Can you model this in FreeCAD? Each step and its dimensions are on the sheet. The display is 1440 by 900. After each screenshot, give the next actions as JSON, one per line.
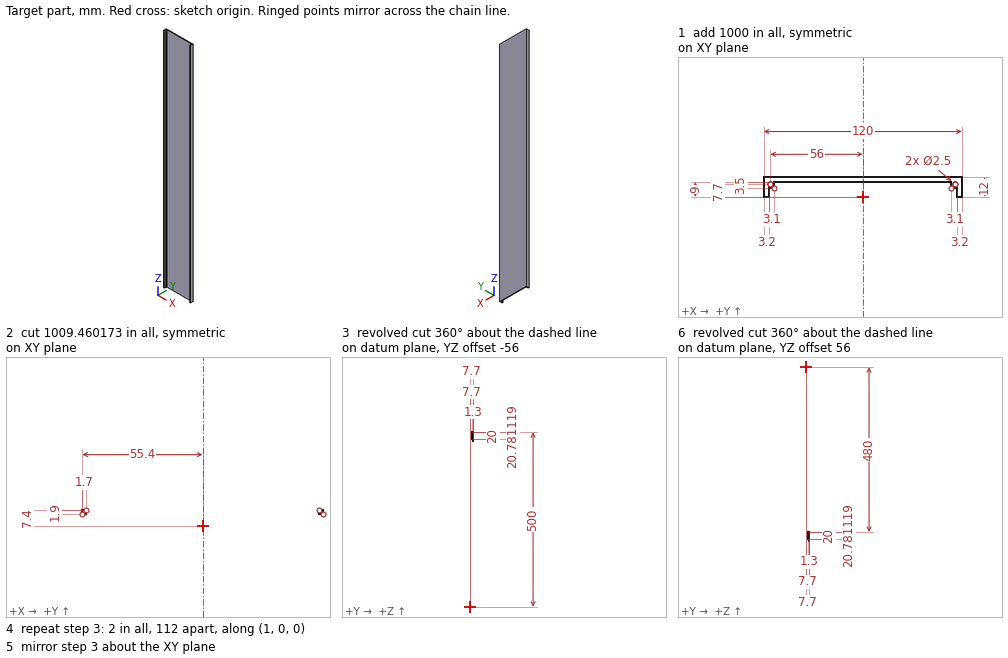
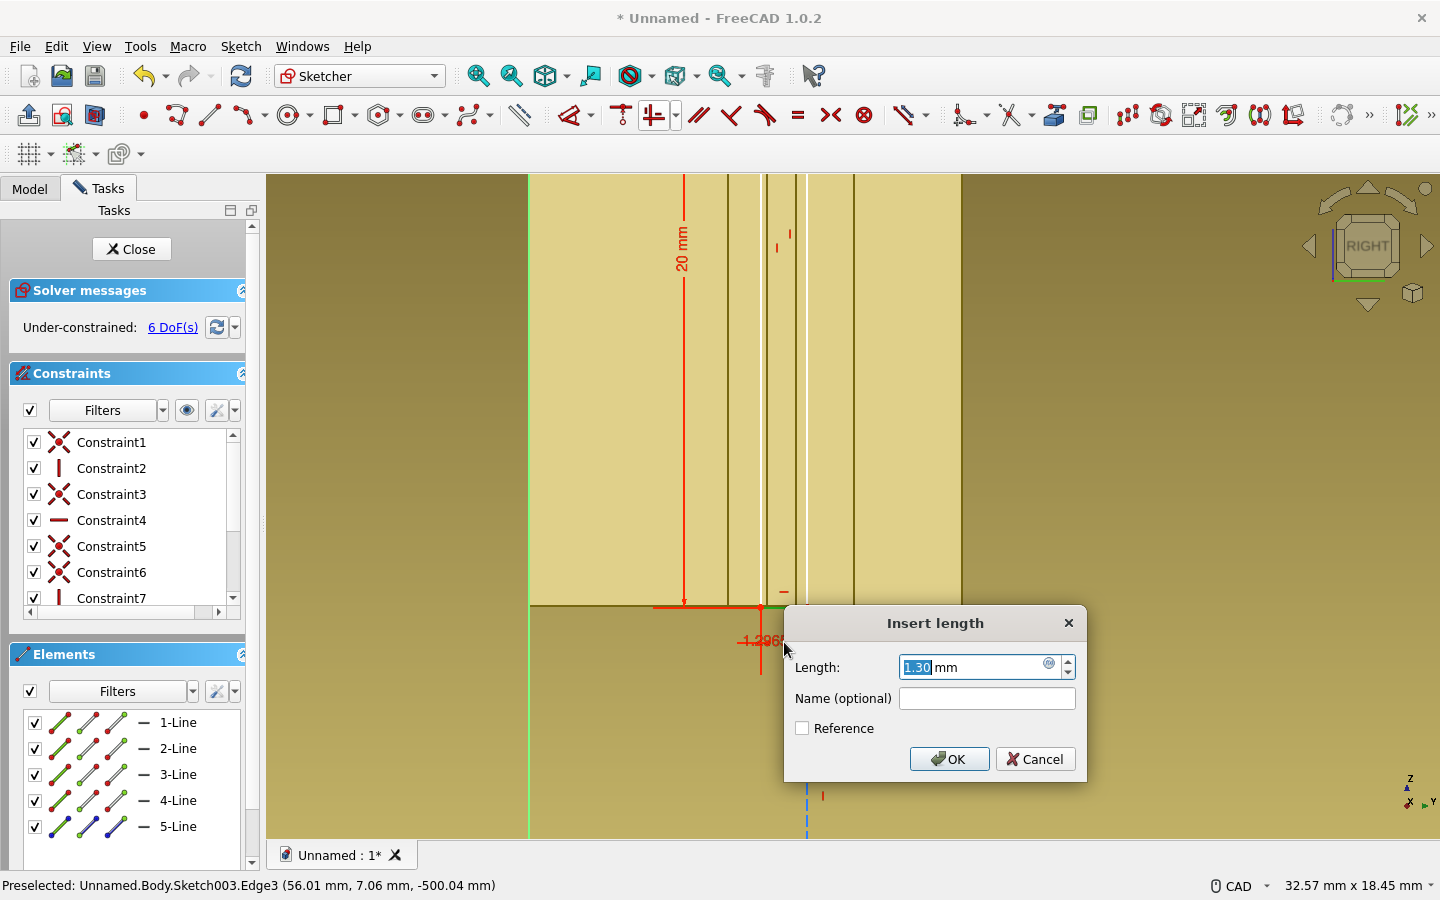
{"action": "type", "text": "1.3"}
{"action": "key", "text": "Return"}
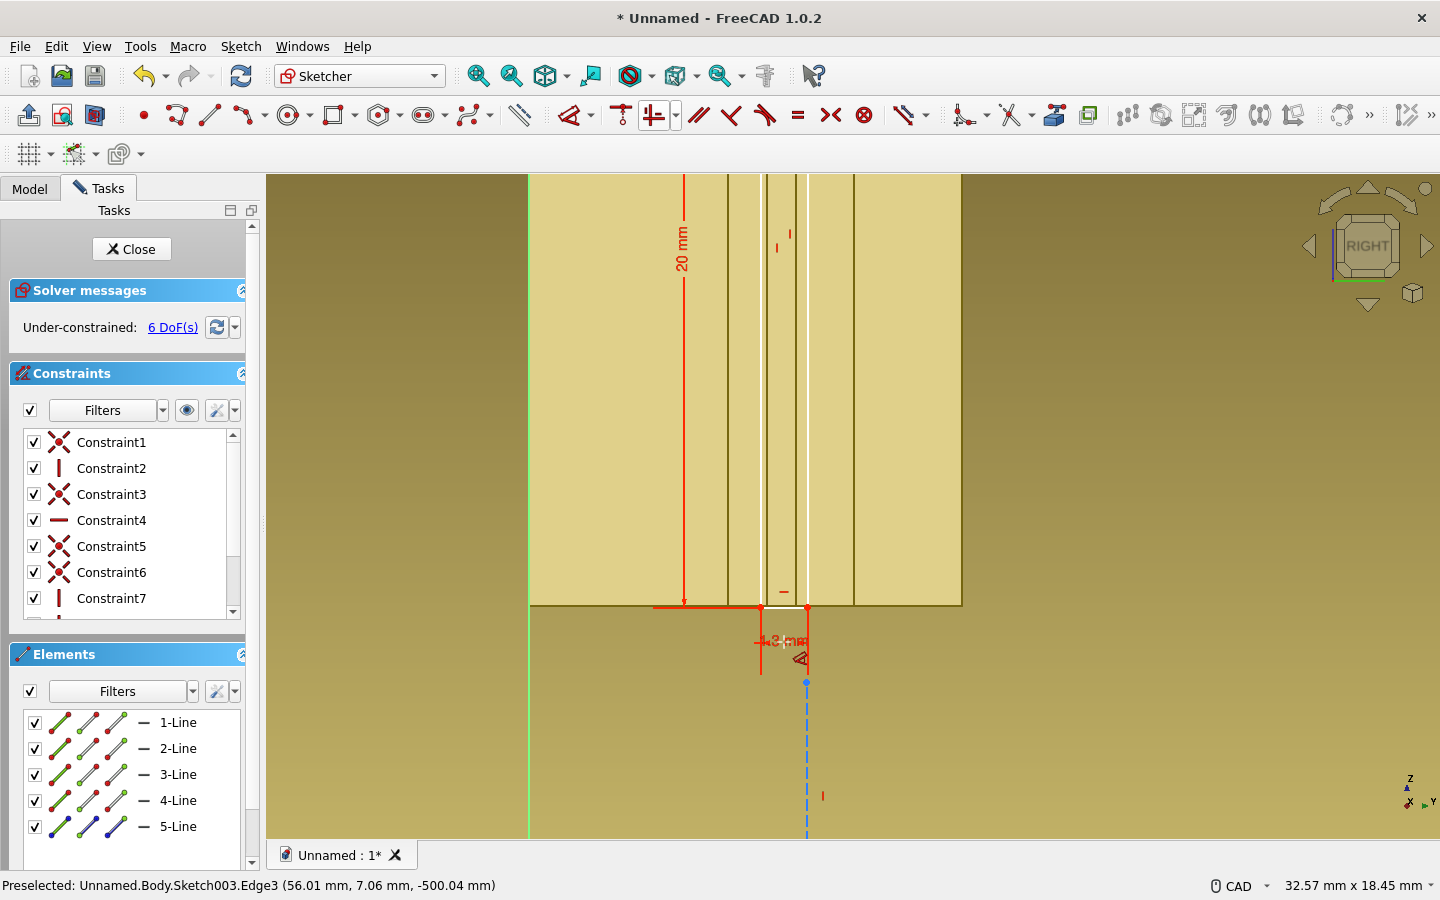
{"action": "scroll", "coordinate": [785, 608], "scroll_direction": "down", "scroll_amount": 4}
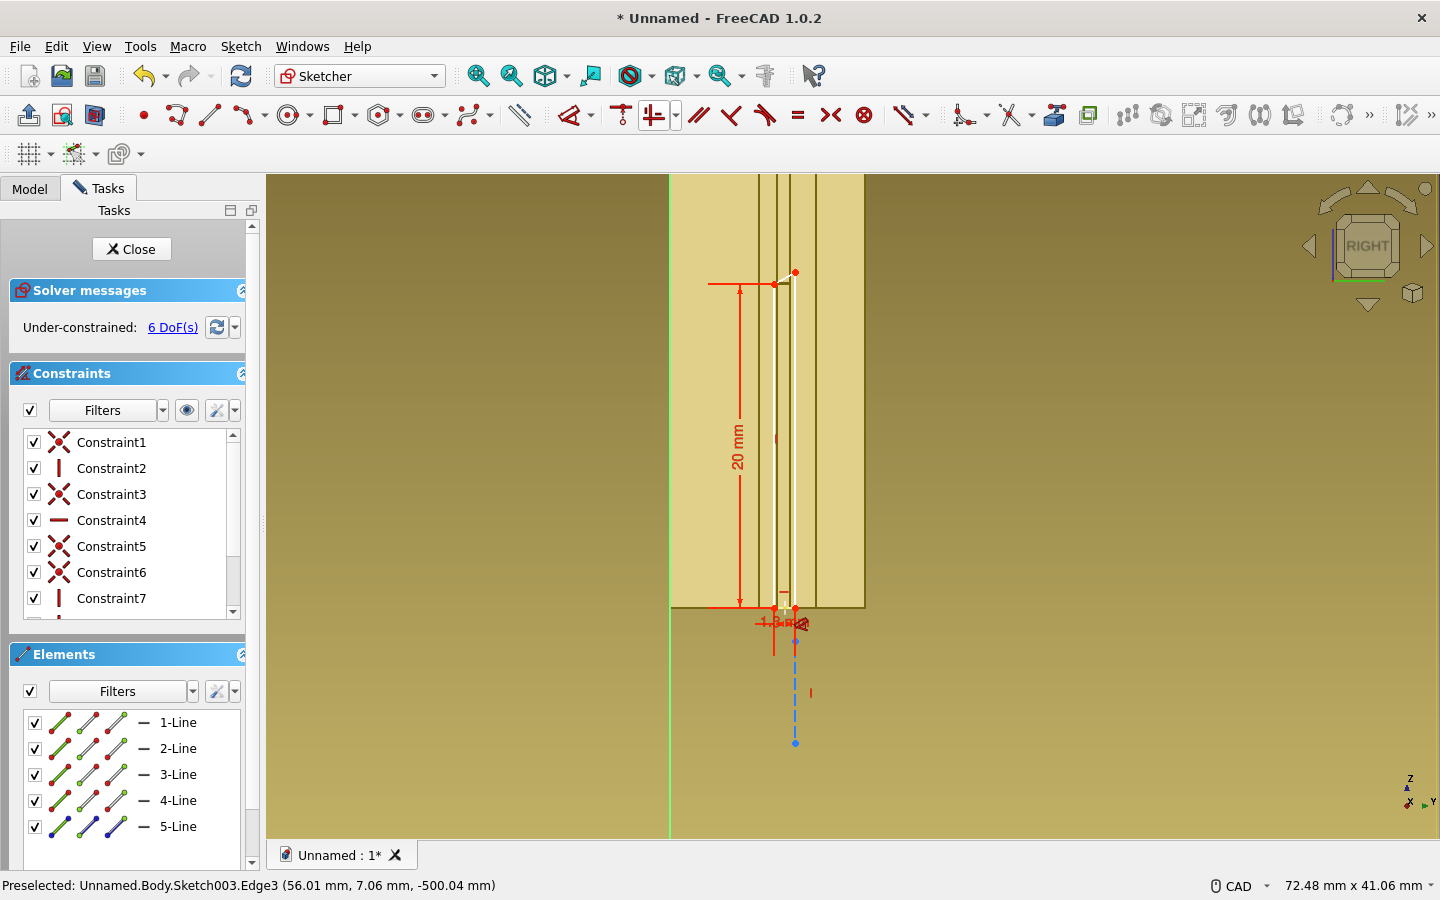
{"action": "left_click", "coordinate": [795, 272]}
{"action": "left_click", "coordinate": [733, 306]}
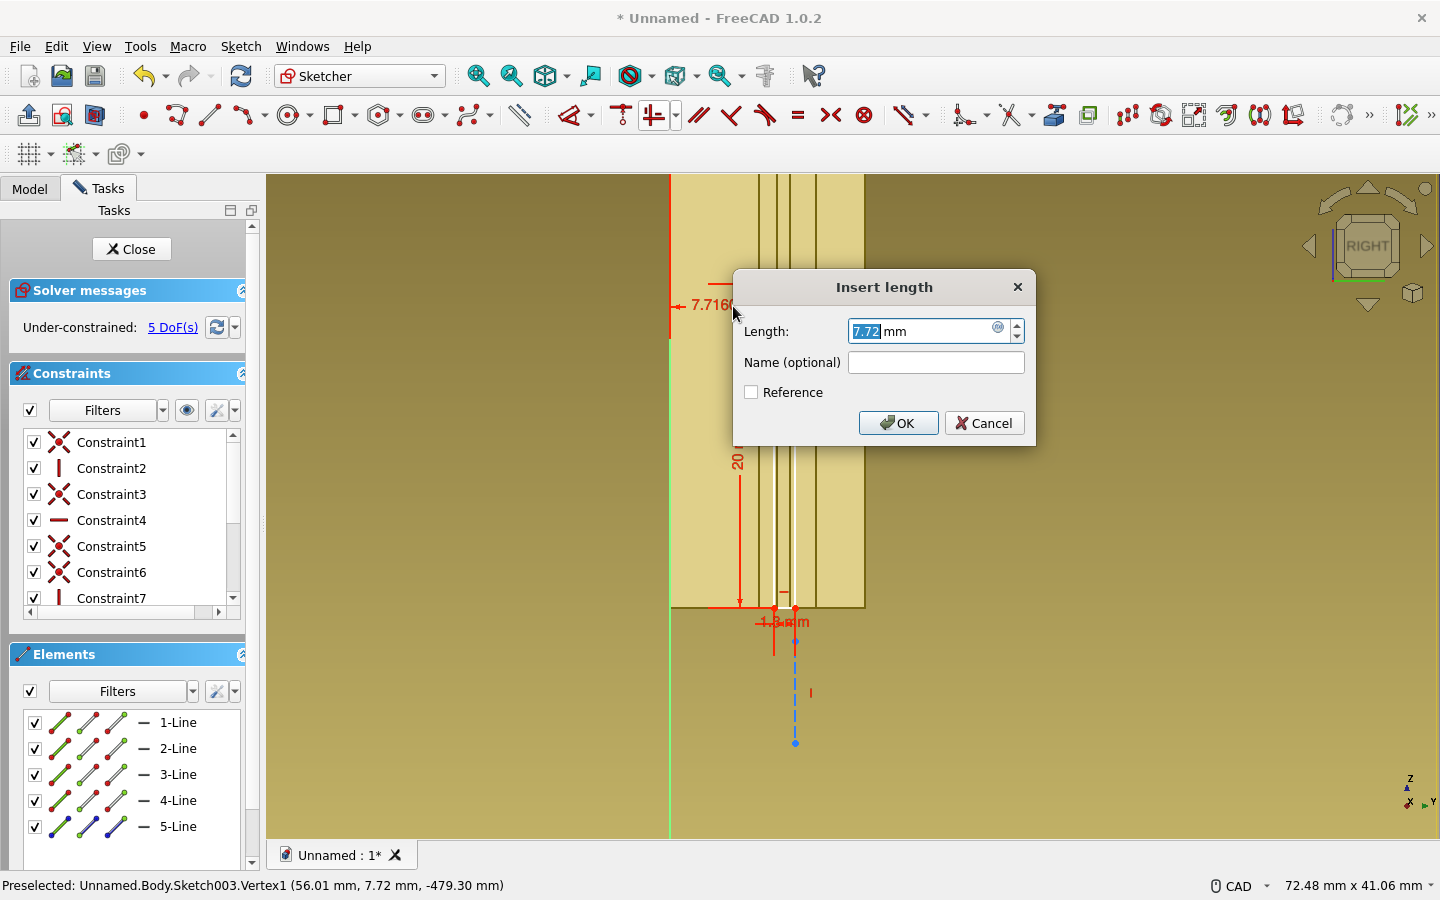
{"action": "type", "text": "7.7"}
{"action": "key", "text": "Return"}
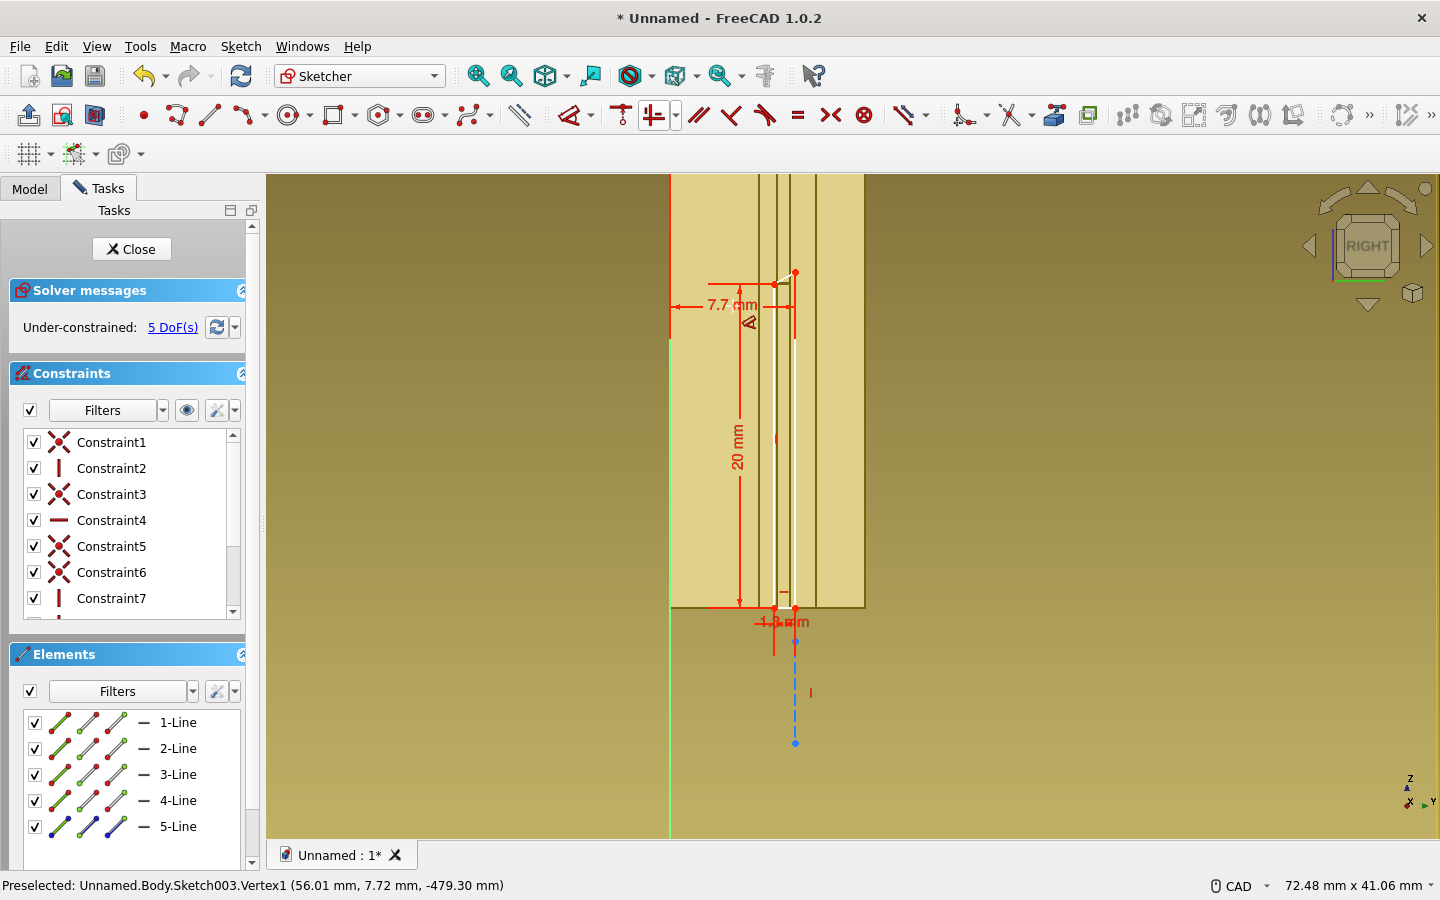
{"action": "left_click", "coordinate": [774, 284]}
{"action": "left_click", "coordinate": [636, 243]}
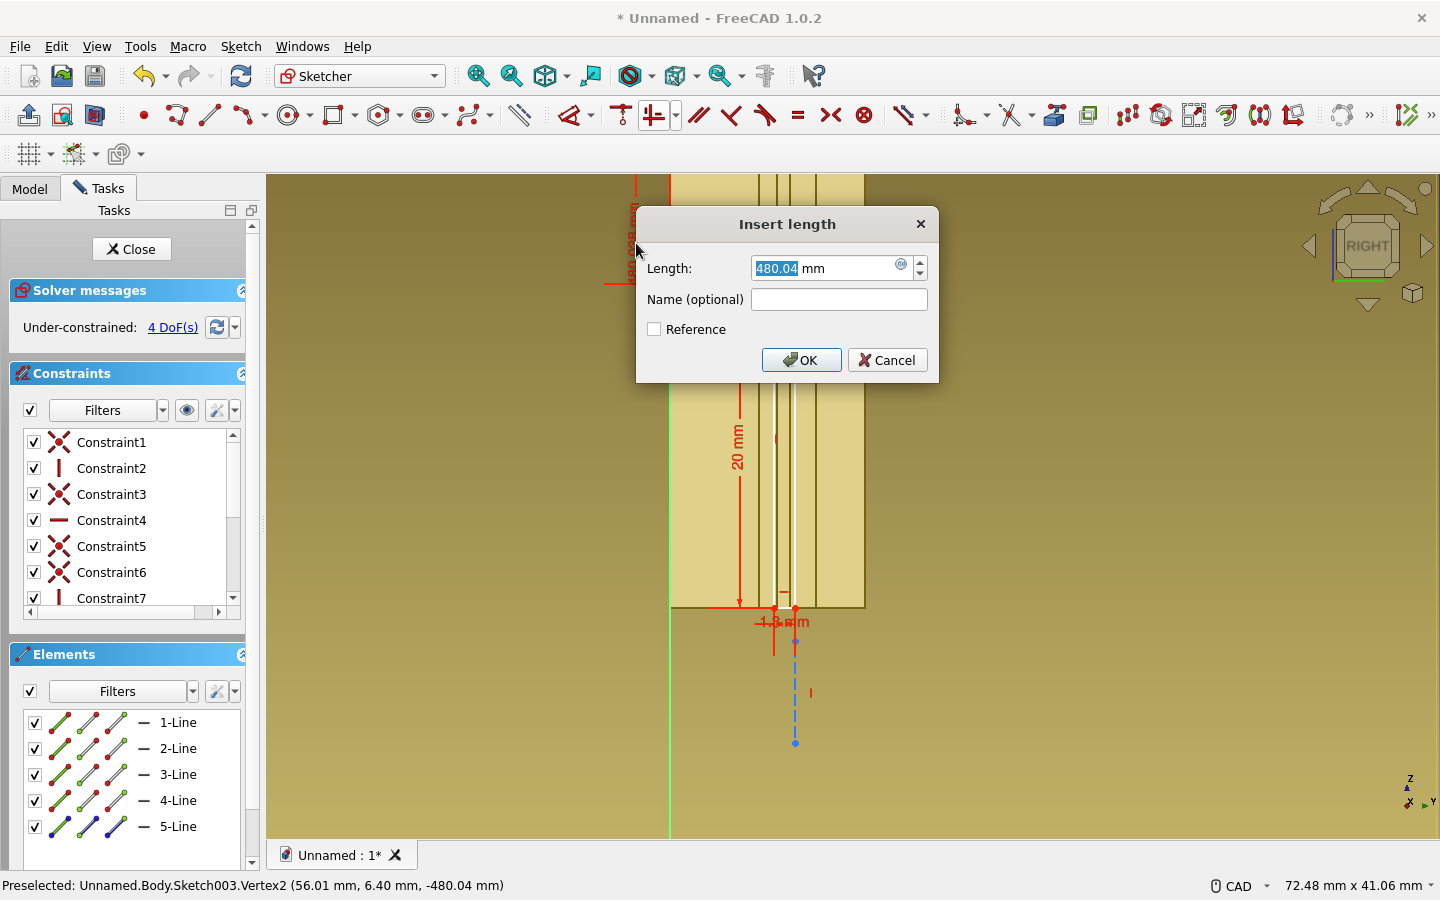
{"action": "type", "text": "480"}
{"action": "key", "text": "Return"}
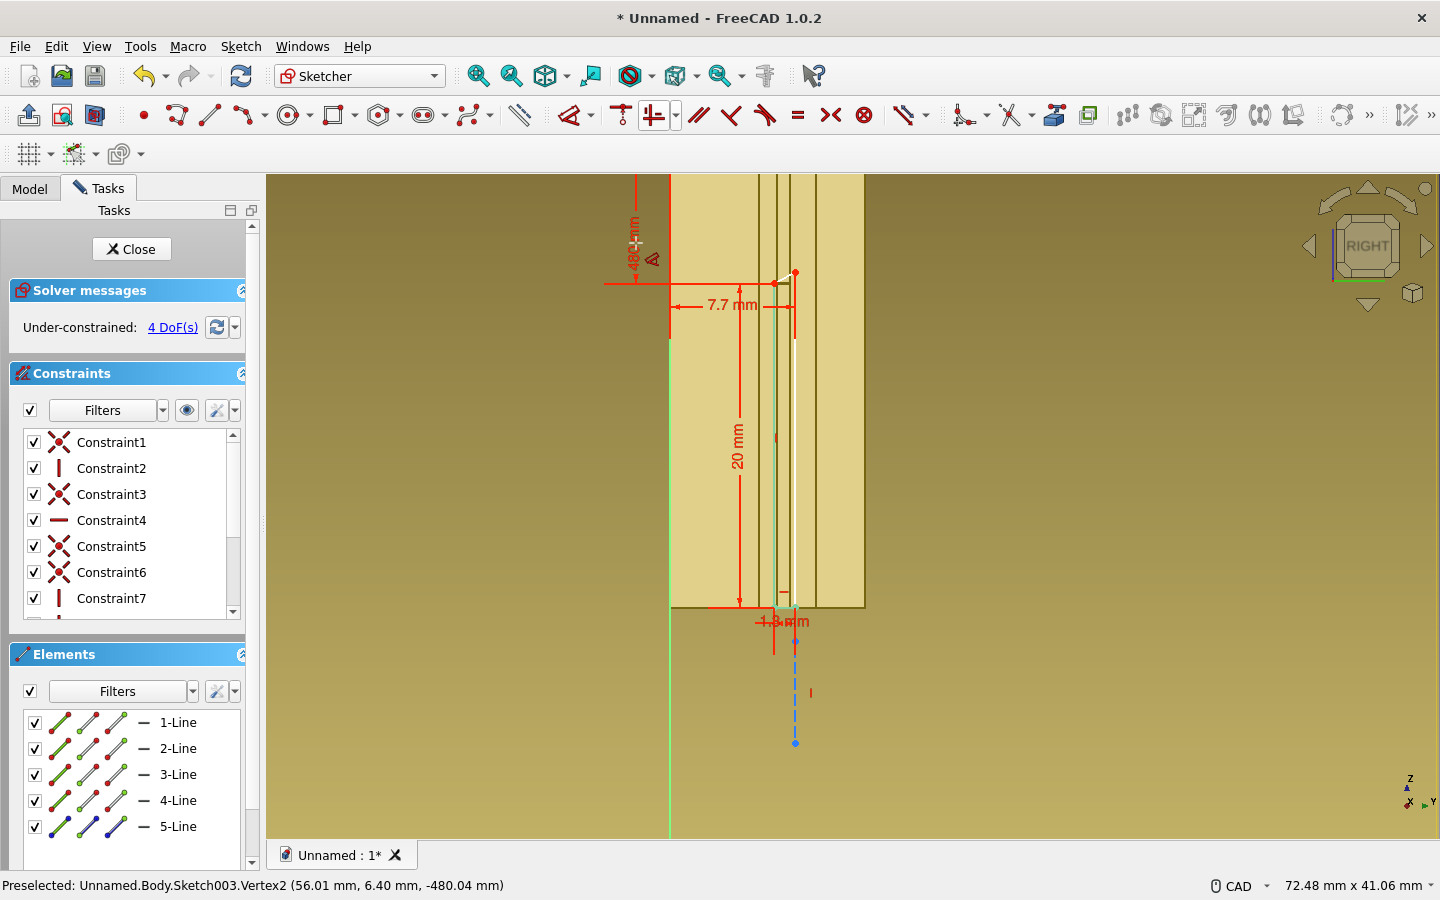
{"action": "left_click", "coordinate": [795, 642]}
{"action": "left_click", "coordinate": [733, 676]}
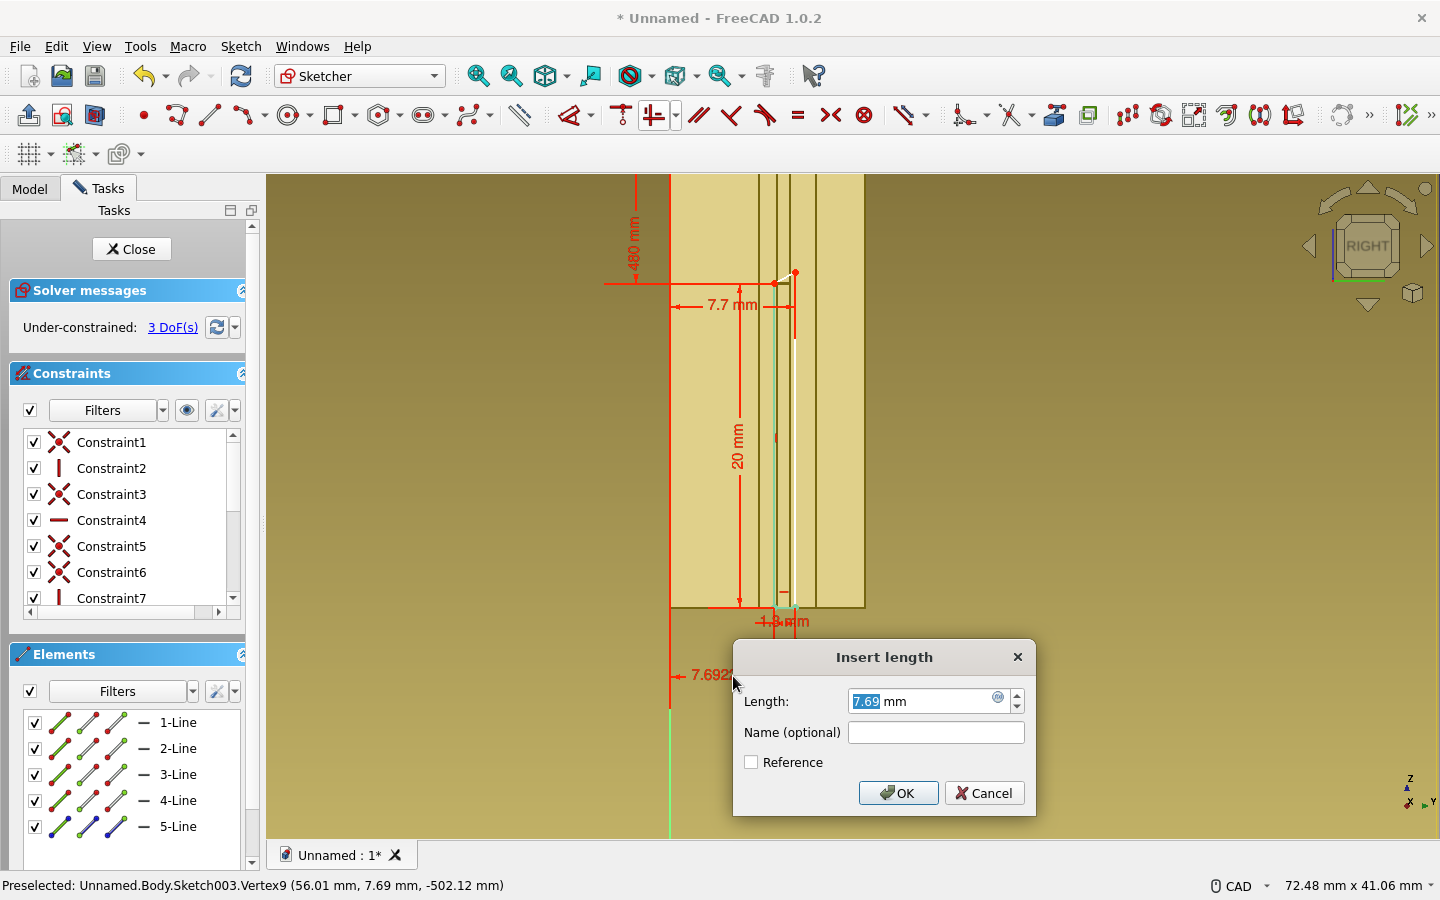
{"action": "type", "text": "7.7"}
{"action": "key", "text": "Return"}